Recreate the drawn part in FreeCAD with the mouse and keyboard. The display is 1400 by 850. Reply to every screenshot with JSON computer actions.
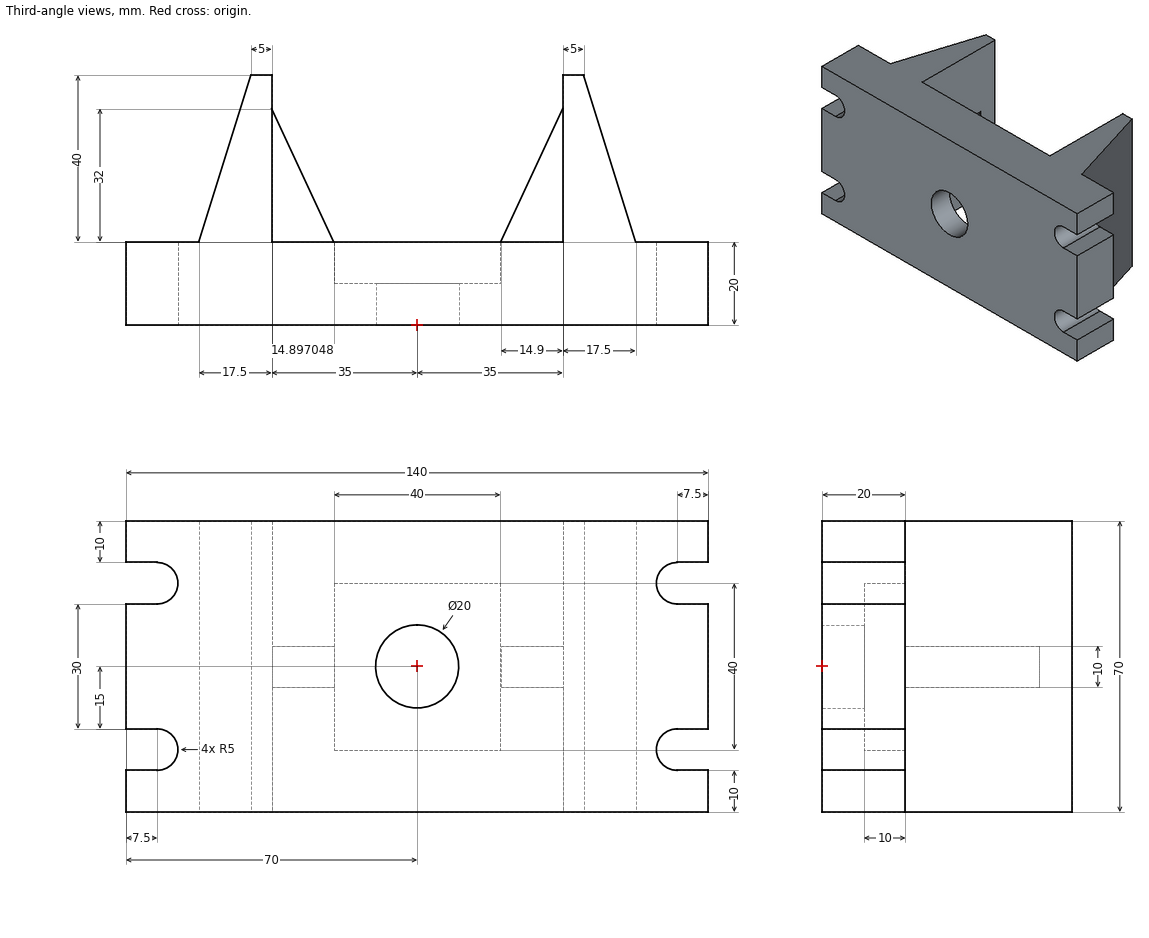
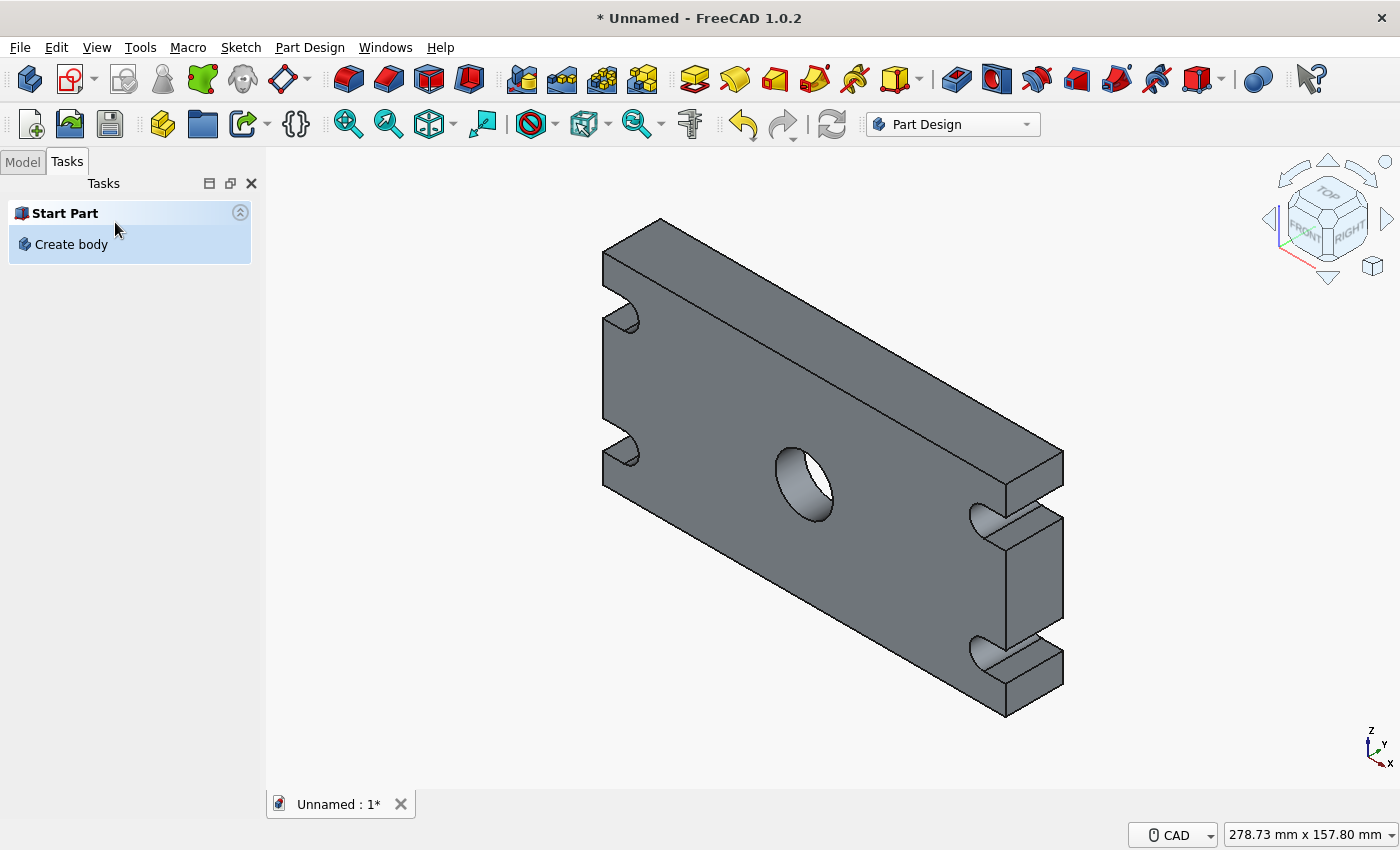
{"action": "left_click", "coordinate": [948, 417]}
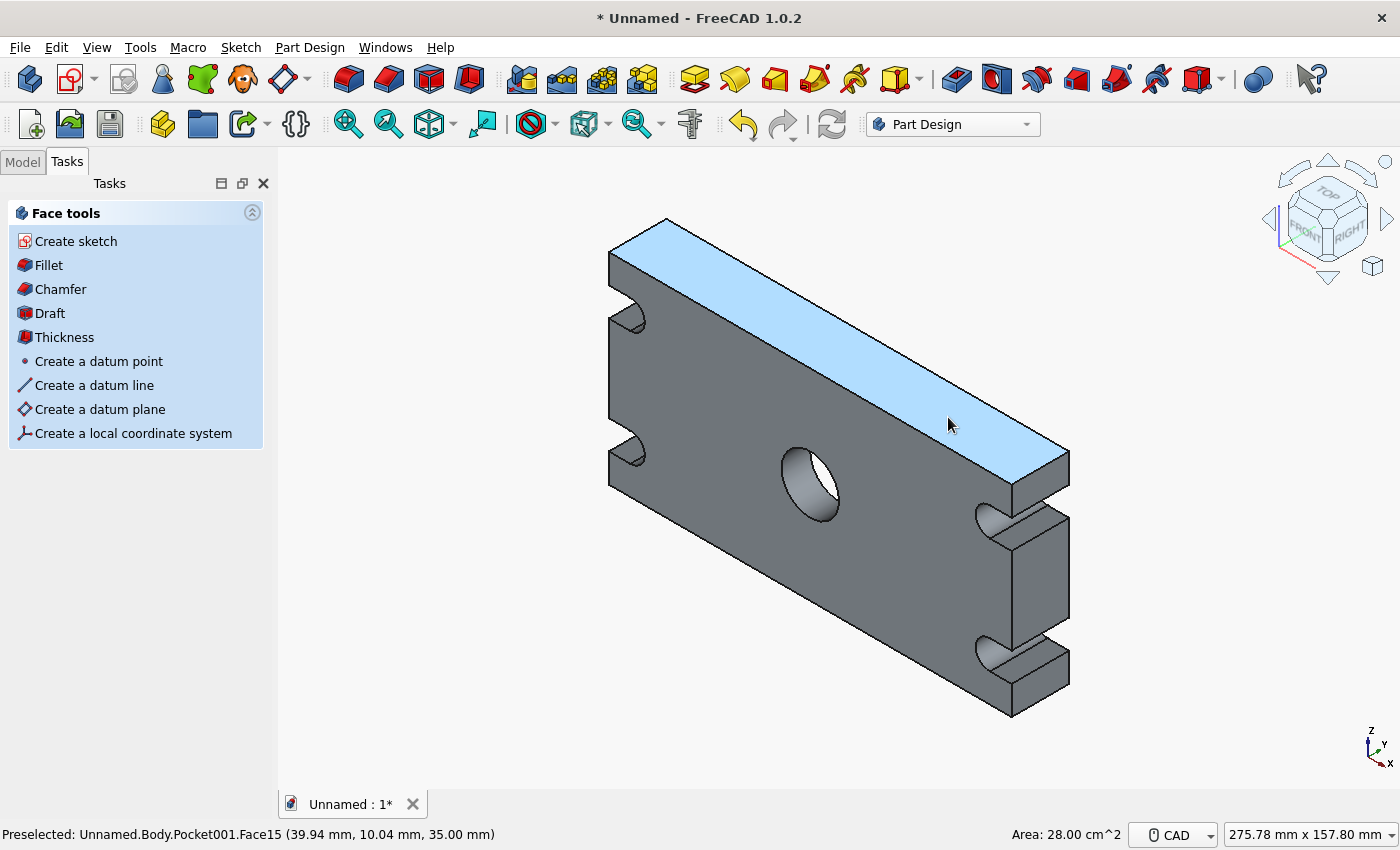
{"action": "left_click", "coordinate": [70, 80]}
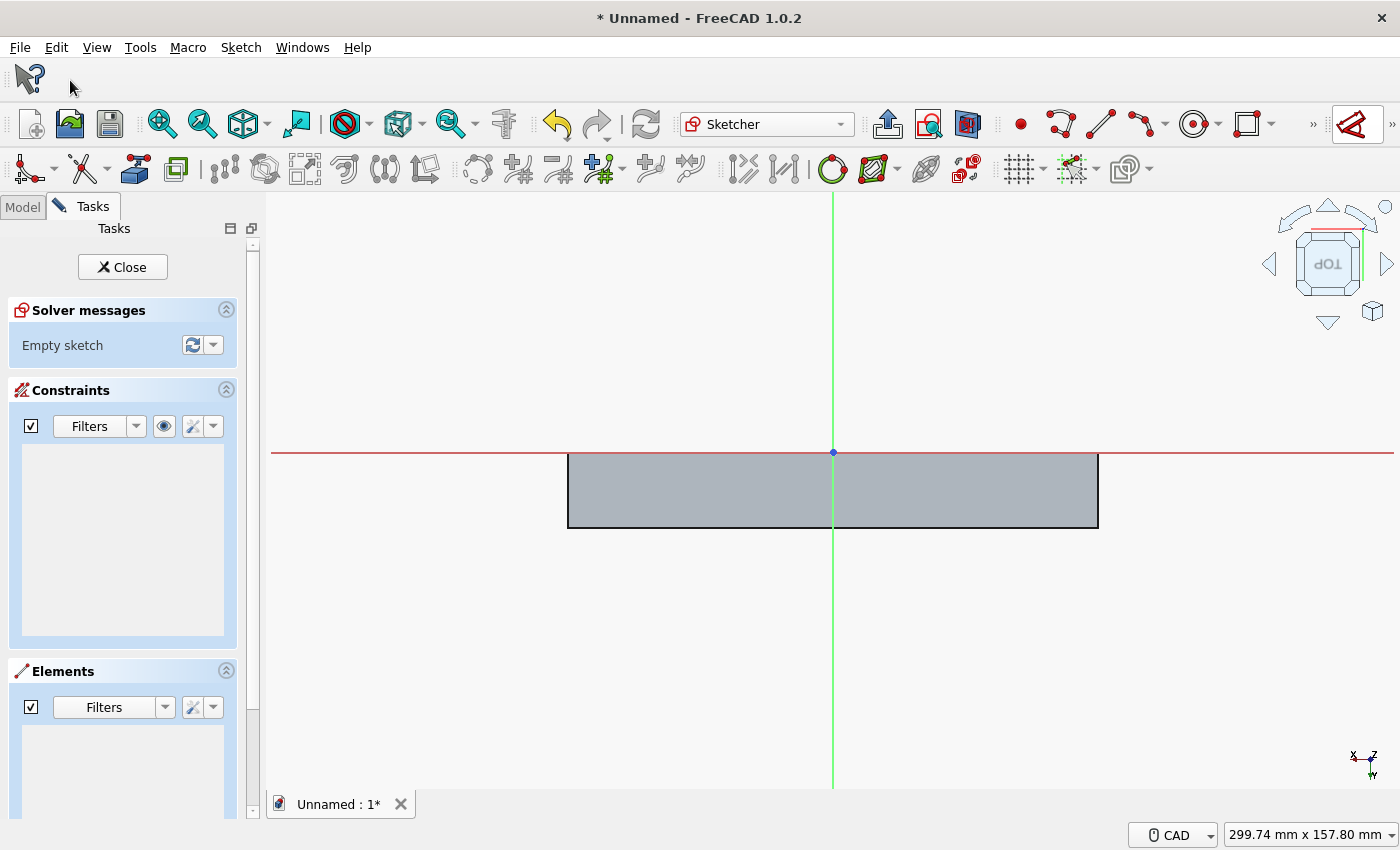
{"action": "scroll", "coordinate": [916, 658], "scroll_direction": "up", "scroll_amount": 3}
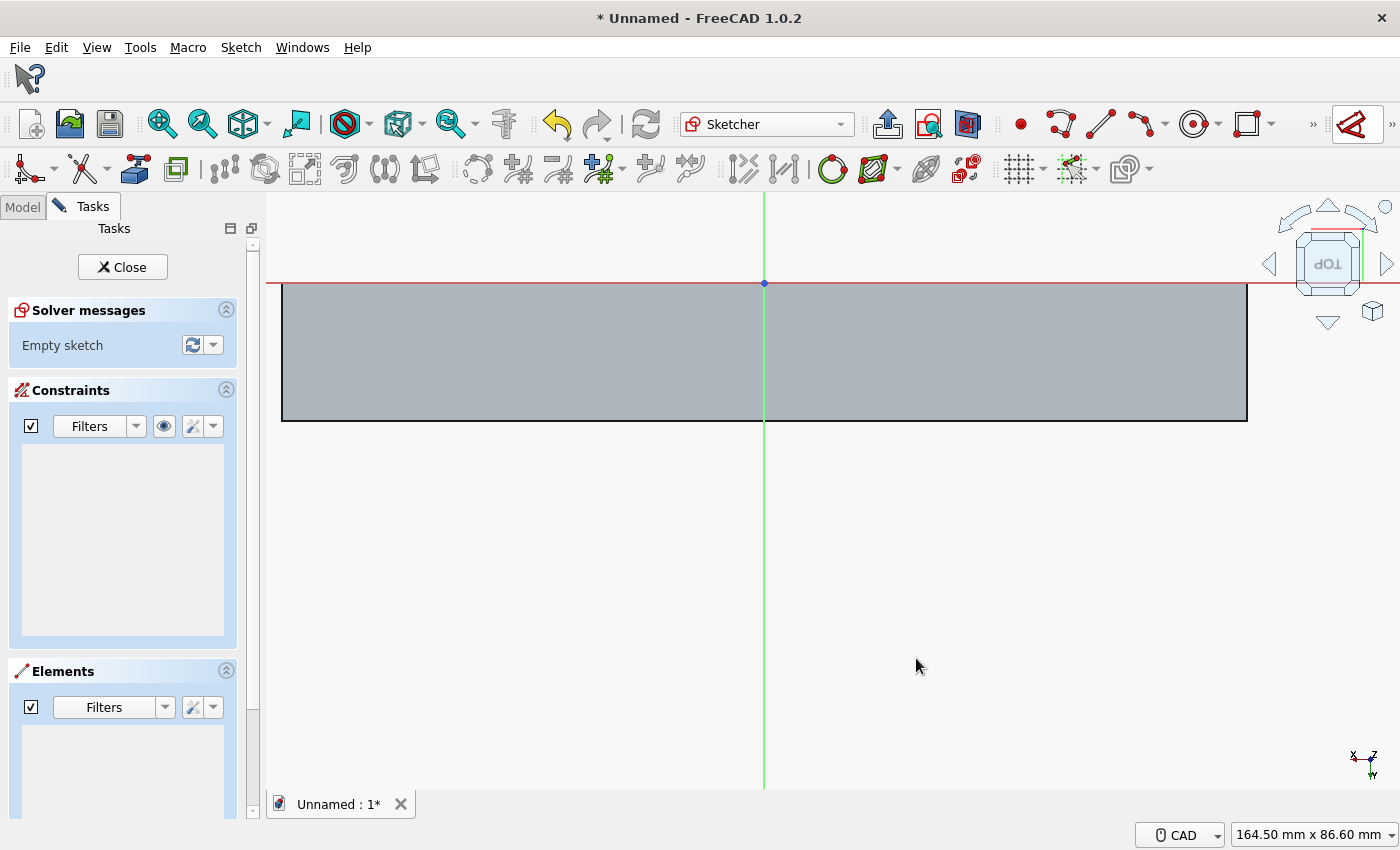
{"action": "left_click", "coordinate": [1062, 124]}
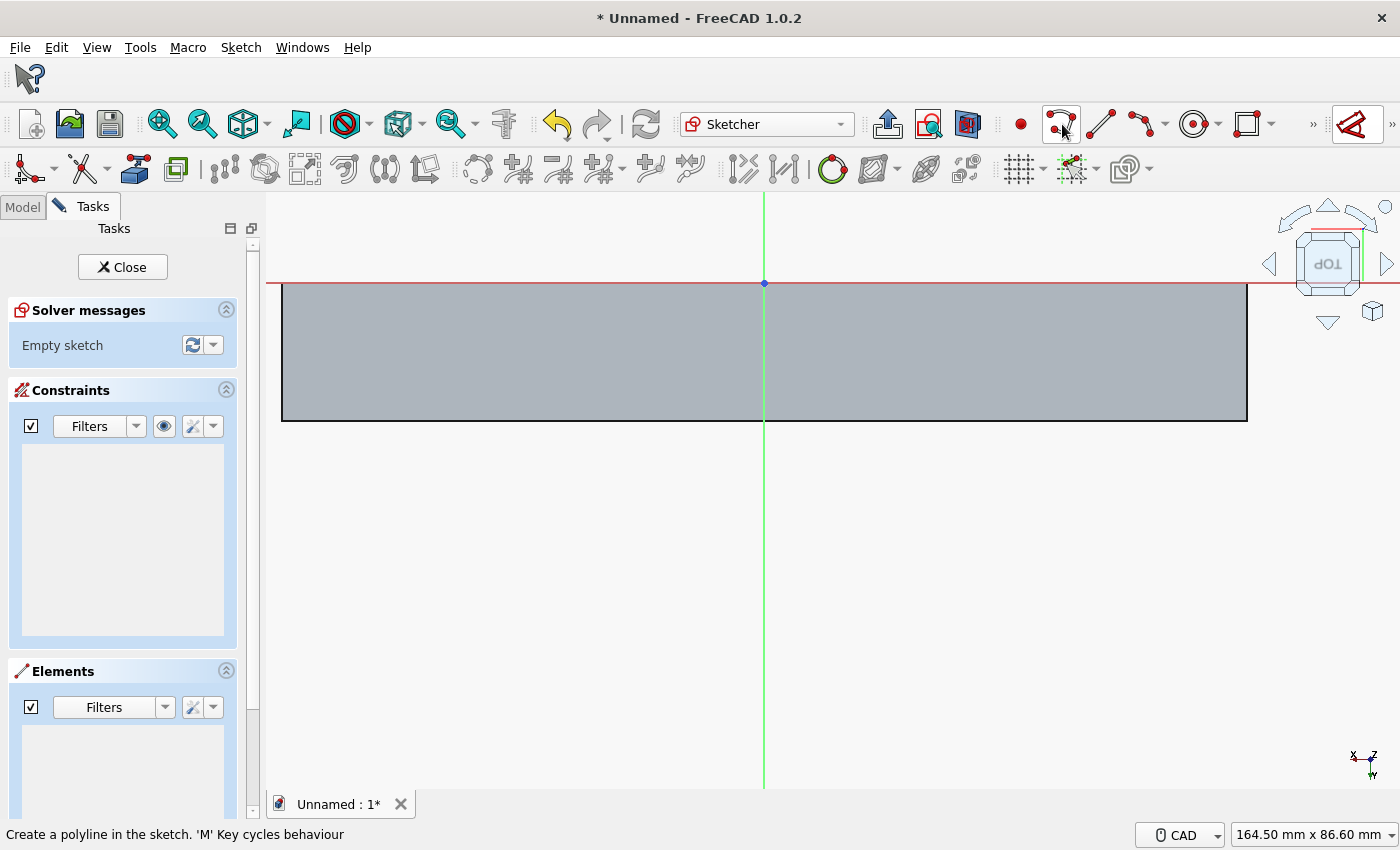
{"action": "left_click", "coordinate": [1006, 421]}
{"action": "left_click", "coordinate": [1006, 697]}
{"action": "left_click", "coordinate": [1040, 697]}
{"action": "left_click", "coordinate": [1126, 421]}
{"action": "left_click", "coordinate": [1006, 422]}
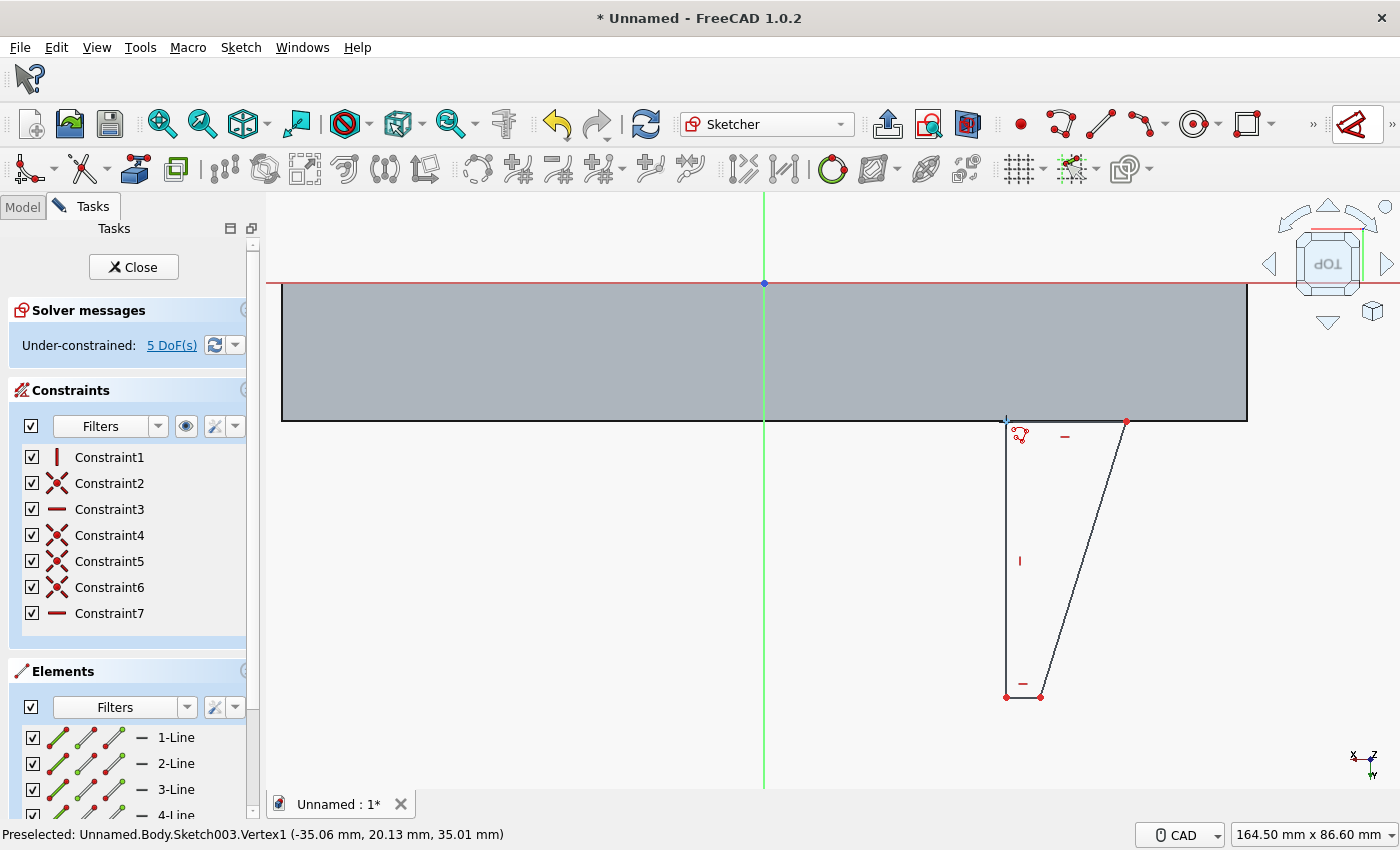
{"action": "left_click", "coordinate": [523, 421]}
{"action": "left_click", "coordinate": [402, 421]}
{"action": "left_click", "coordinate": [489, 697]}
{"action": "left_click", "coordinate": [523, 697]}
{"action": "left_click", "coordinate": [523, 422]}
{"action": "key", "text": "Escape"}
{"action": "key", "text": "Escape"}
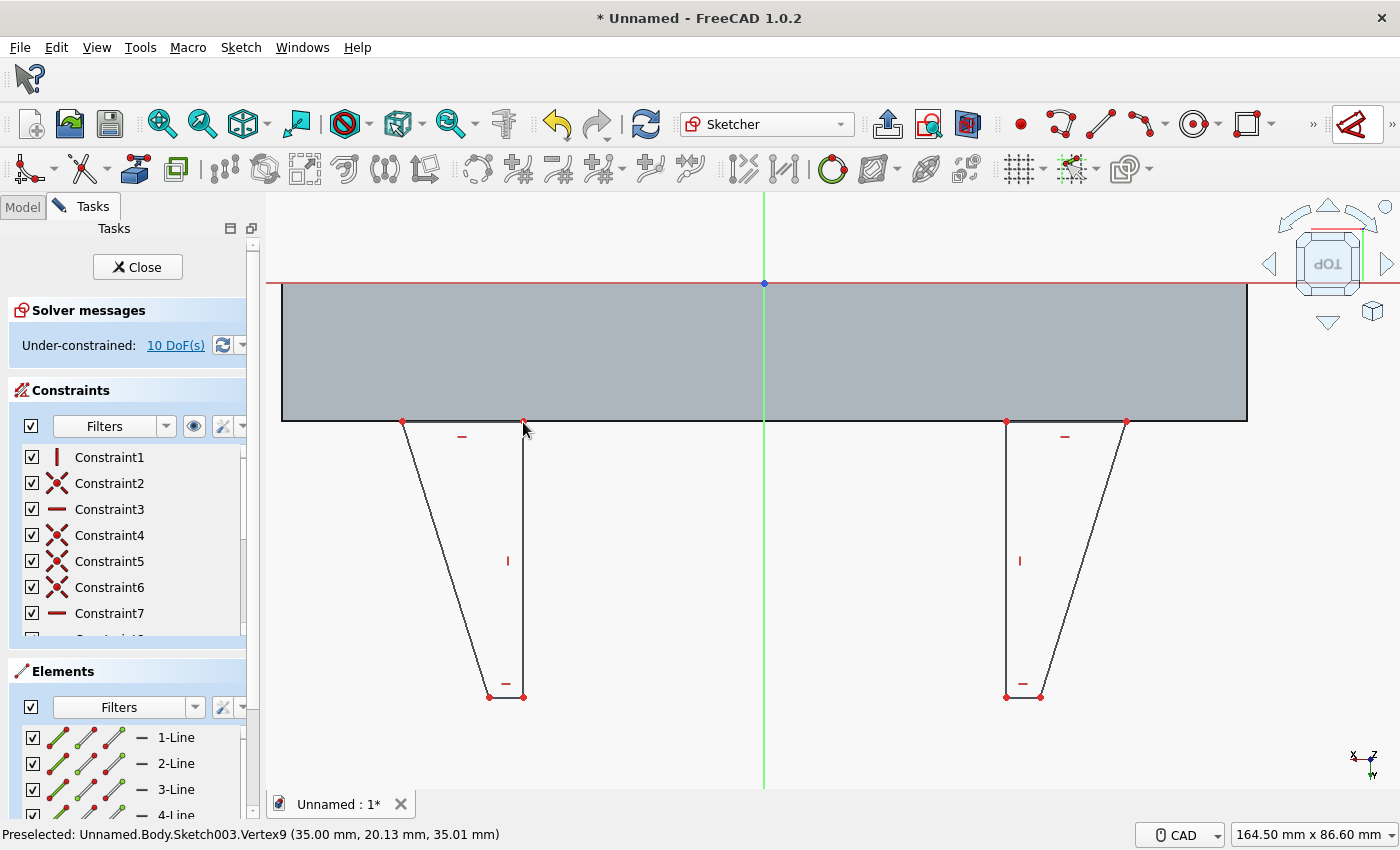
{"action": "scroll", "coordinate": [1016, 698], "scroll_direction": "up", "scroll_amount": 2}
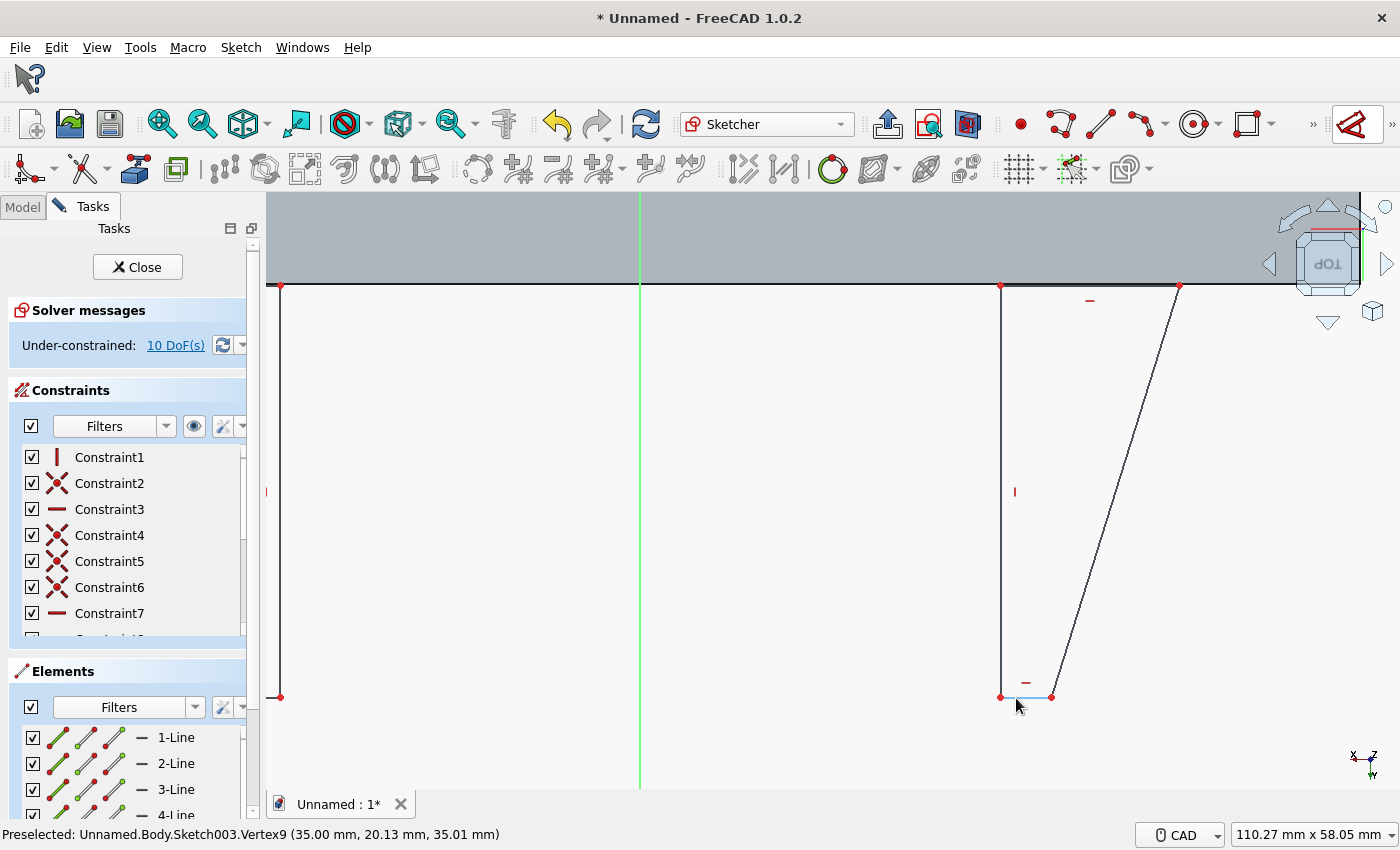
{"action": "left_click", "coordinate": [1016, 698]}